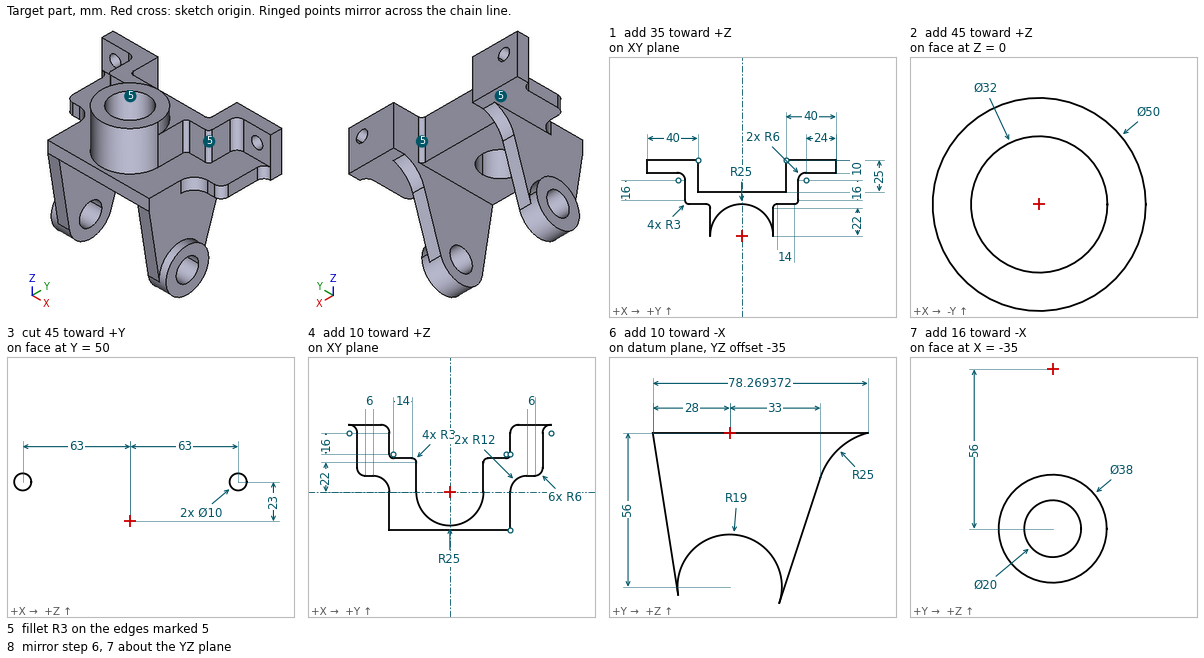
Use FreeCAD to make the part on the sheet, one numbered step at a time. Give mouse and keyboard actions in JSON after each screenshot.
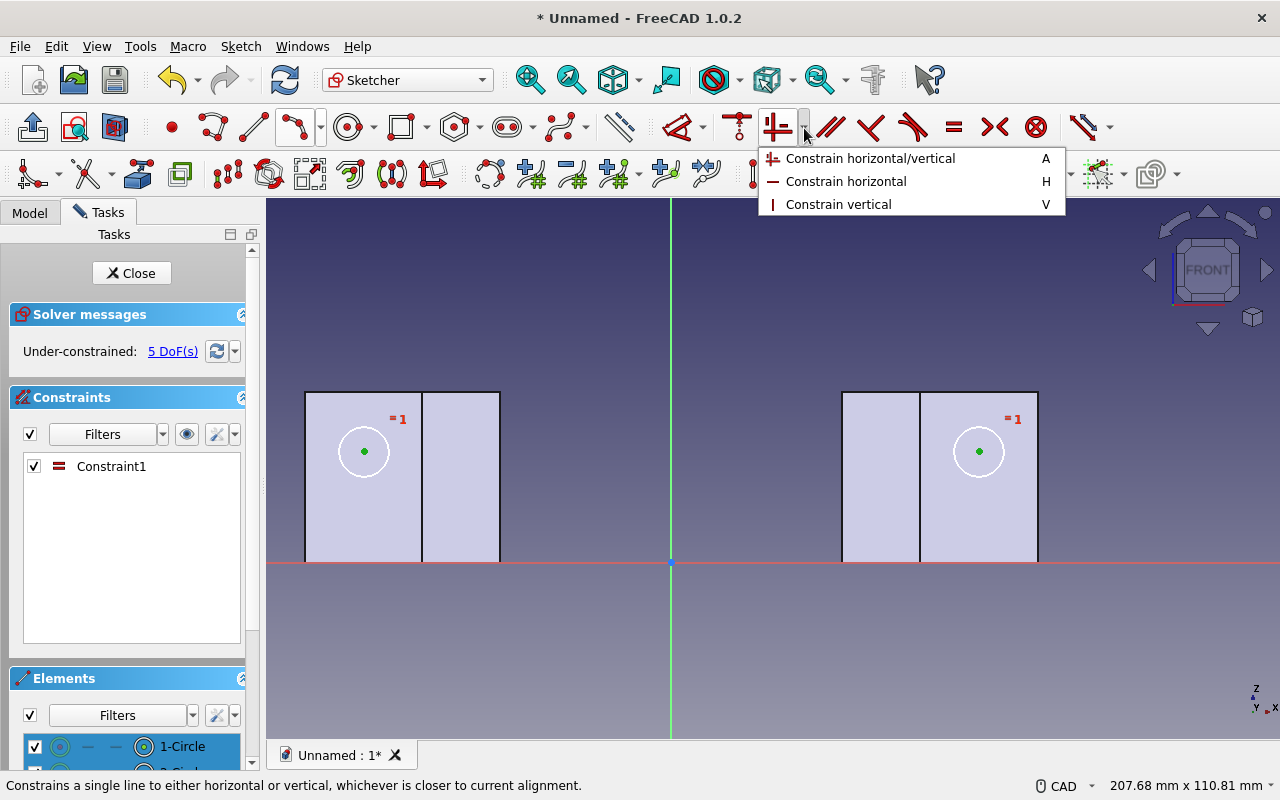
{"action": "left_click", "coordinate": [912, 182]}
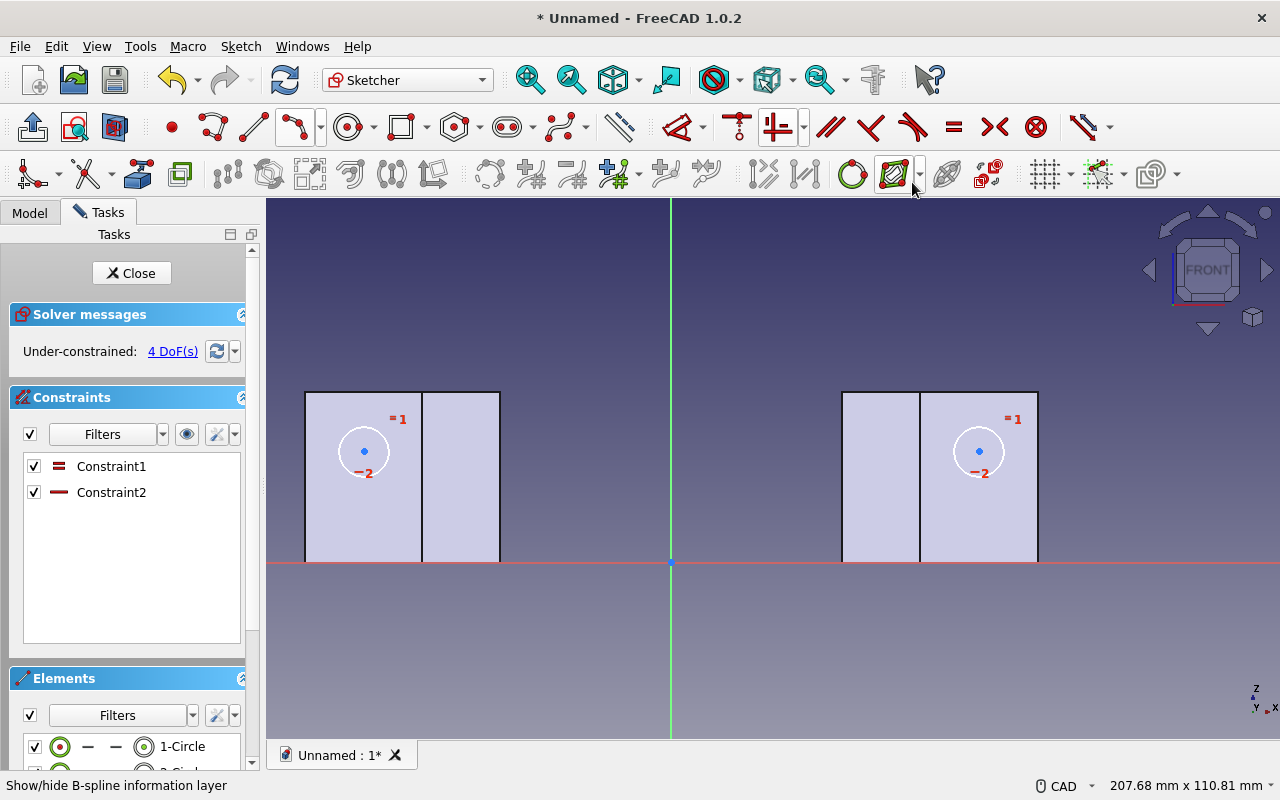
{"action": "left_click", "coordinate": [676, 128]}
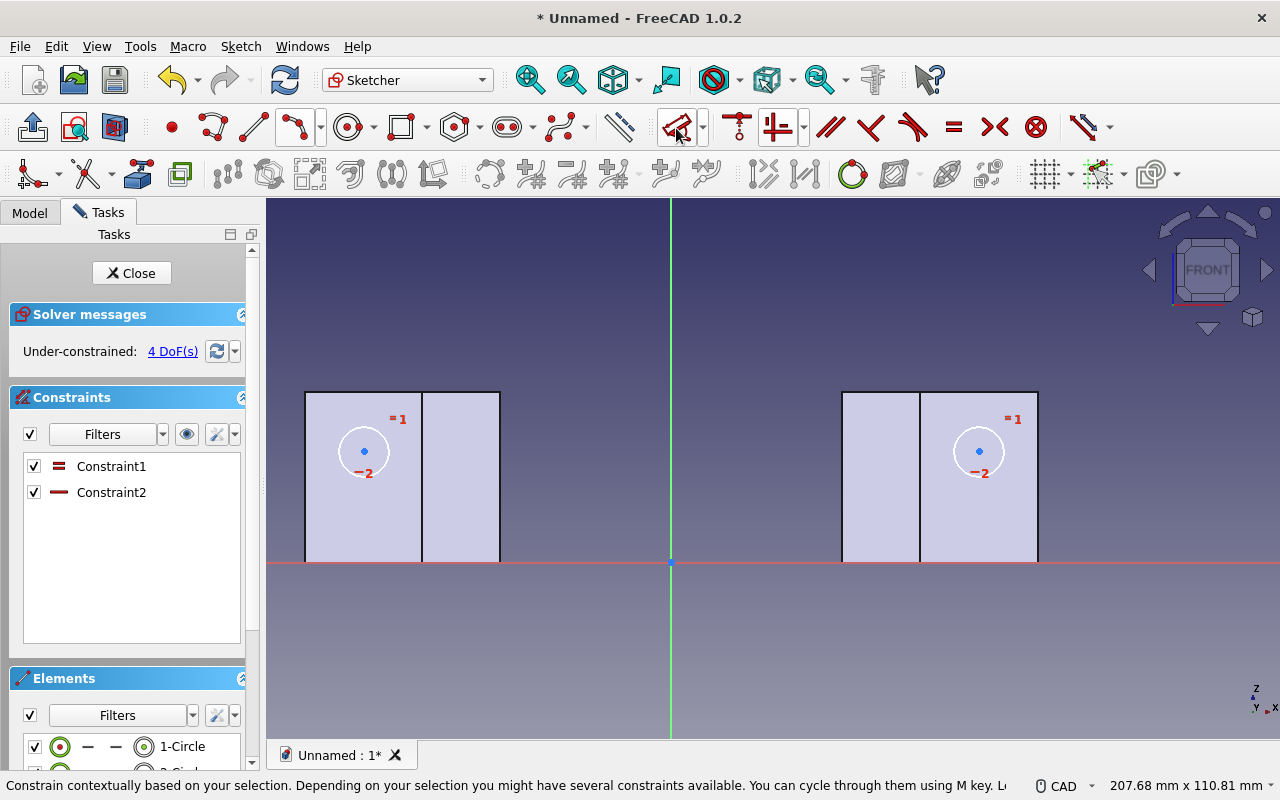
{"action": "left_click", "coordinate": [996, 434]}
{"action": "left_click", "coordinate": [1018, 411]}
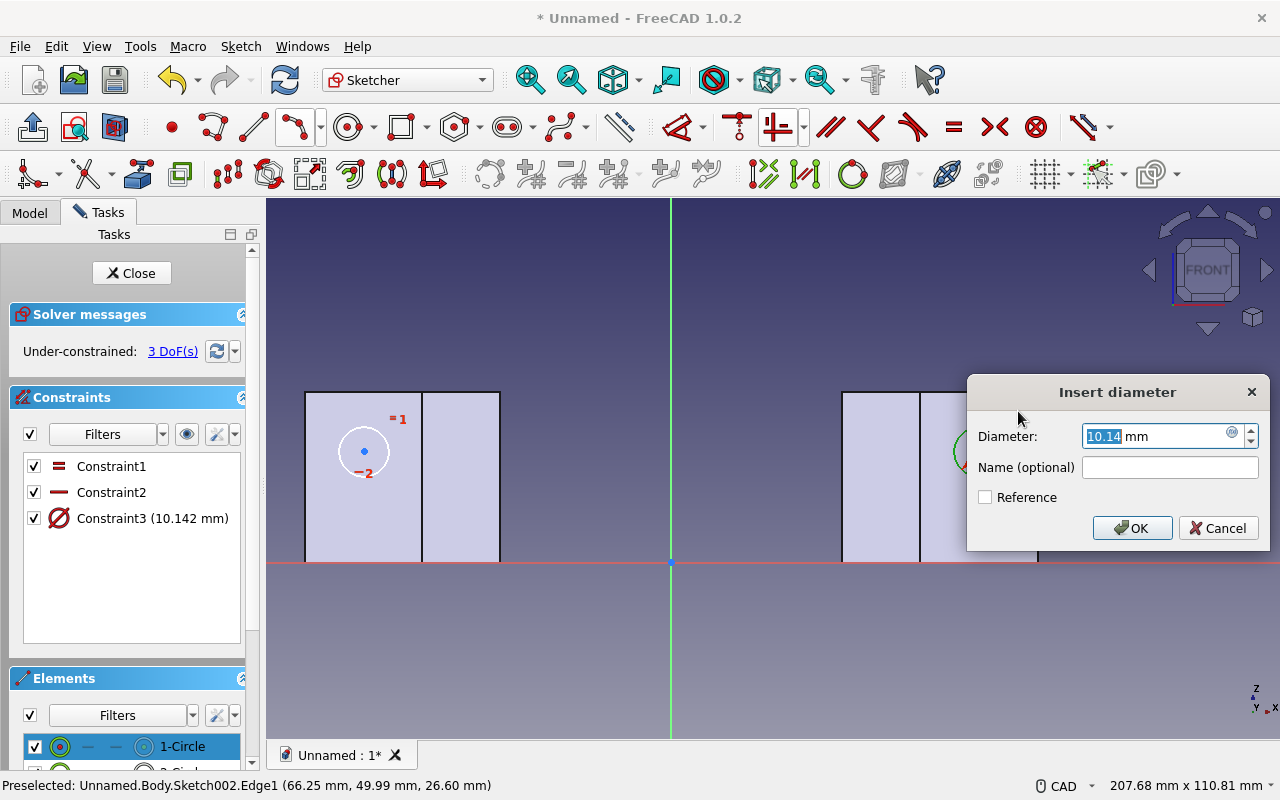
{"action": "type", "text": "10"}
{"action": "key", "text": "Return"}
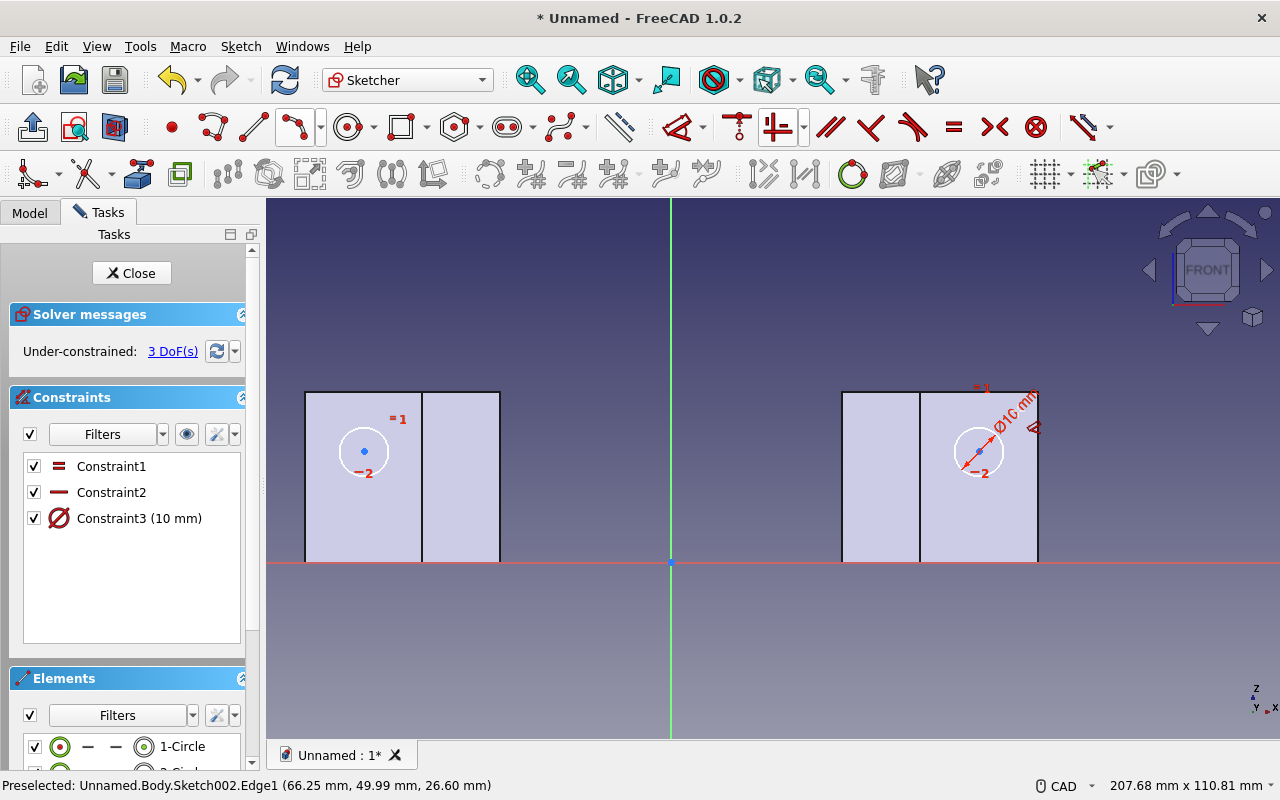
{"action": "left_click", "coordinate": [979, 452]}
{"action": "left_click", "coordinate": [825, 597]}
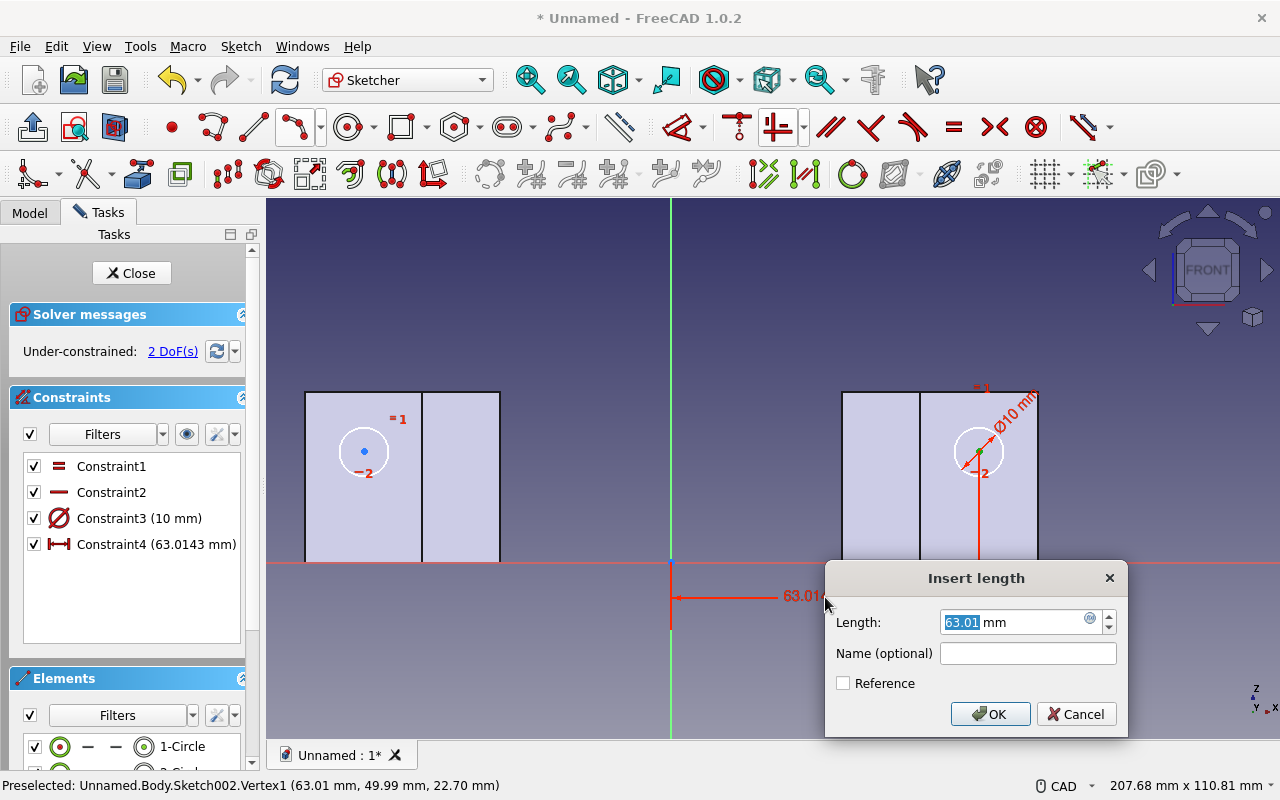
{"action": "type", "text": "63"}
{"action": "key", "text": "Return"}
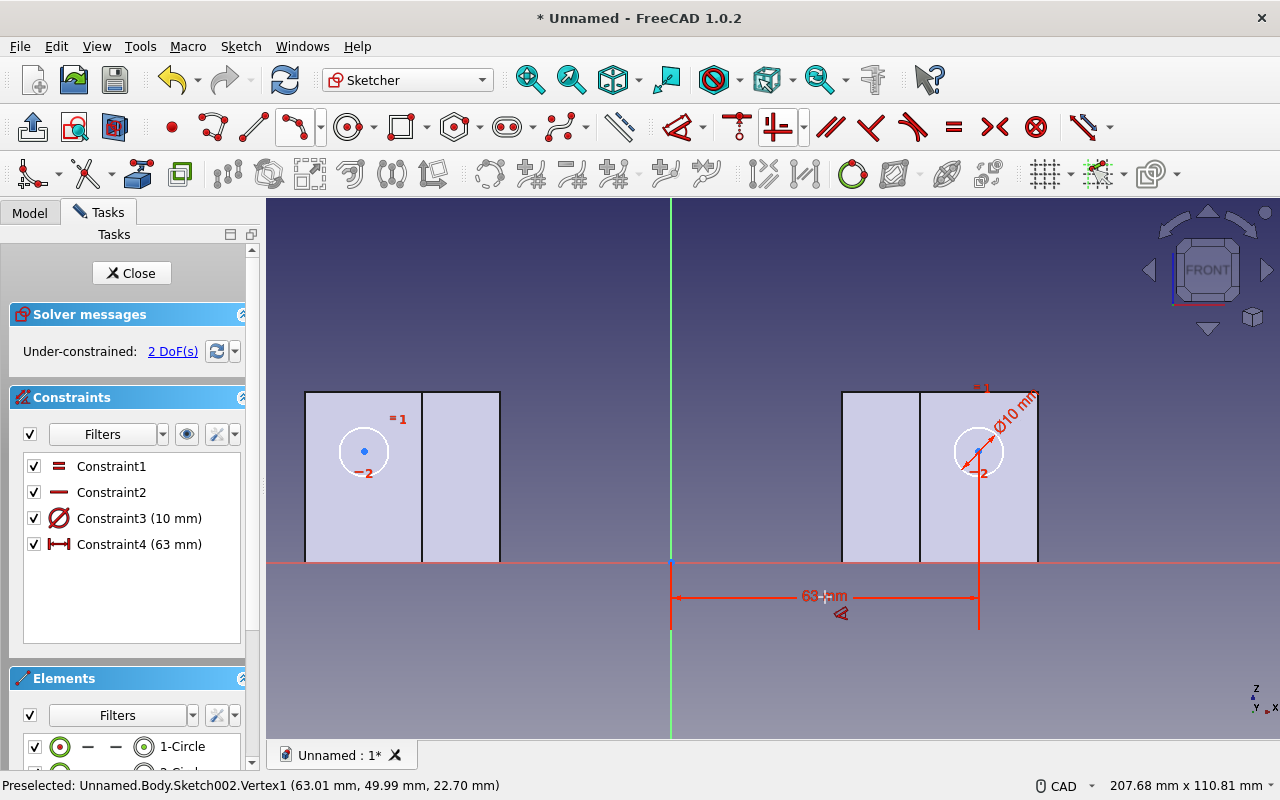
{"action": "left_click", "coordinate": [979, 452]}
{"action": "left_click", "coordinate": [1013, 507]}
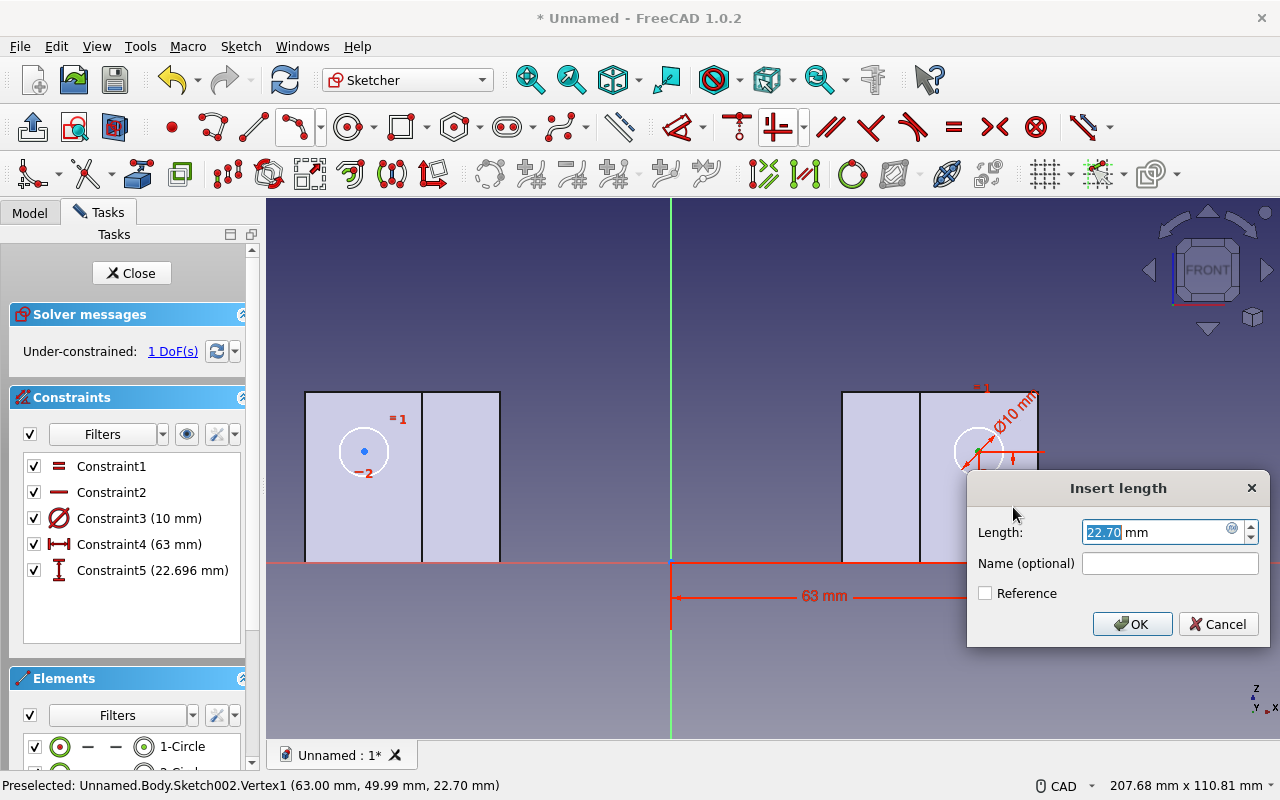
{"action": "type", "text": "23"}
{"action": "key", "text": "Return"}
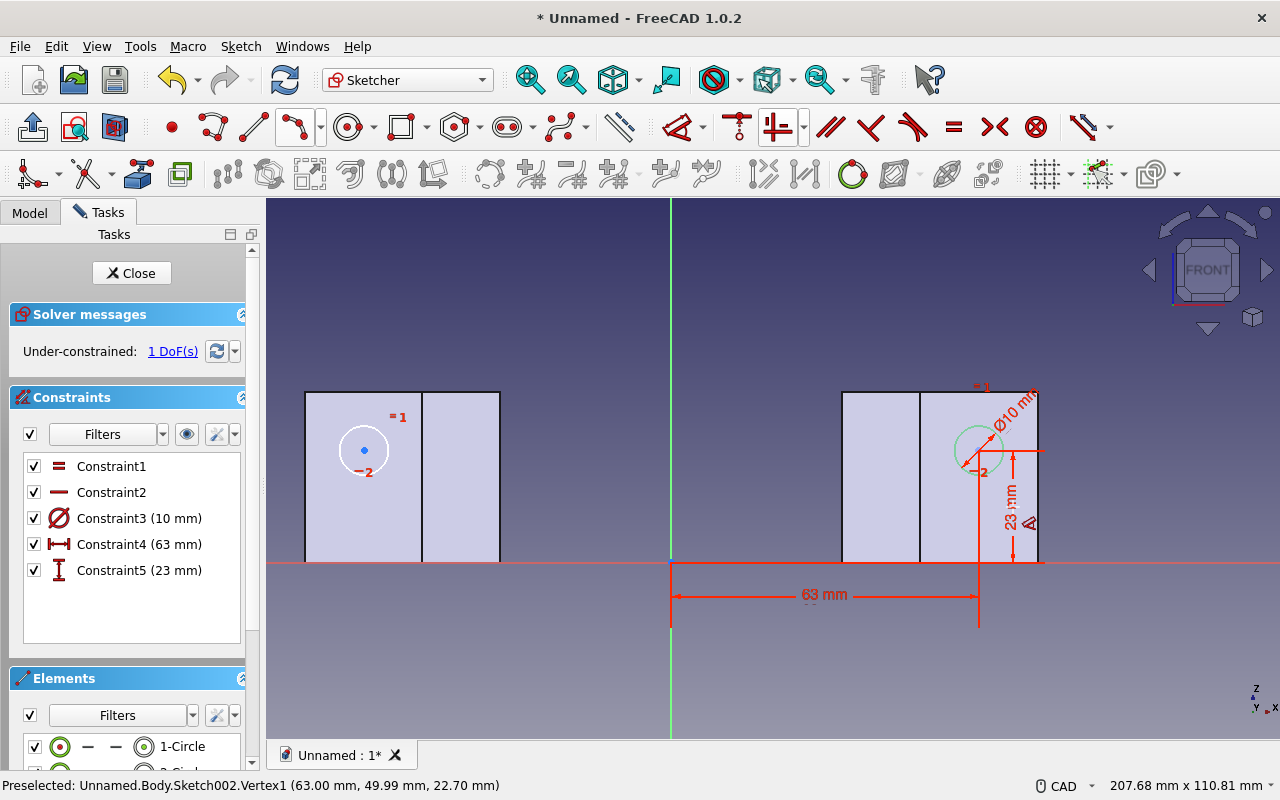
{"action": "left_click", "coordinate": [364, 451]}
{"action": "left_click", "coordinate": [518, 597]}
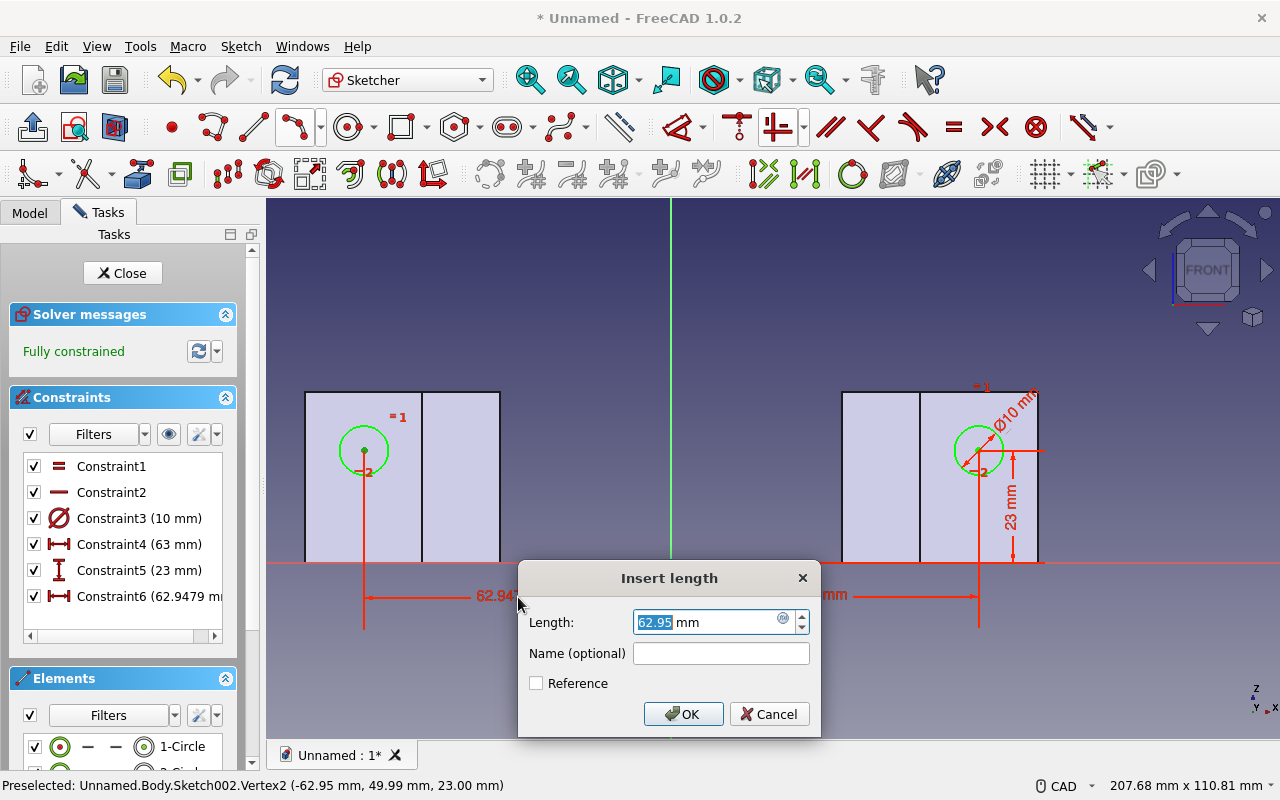
{"action": "type", "text": "63"}
{"action": "key", "text": "Return"}
{"action": "key", "text": "Escape"}